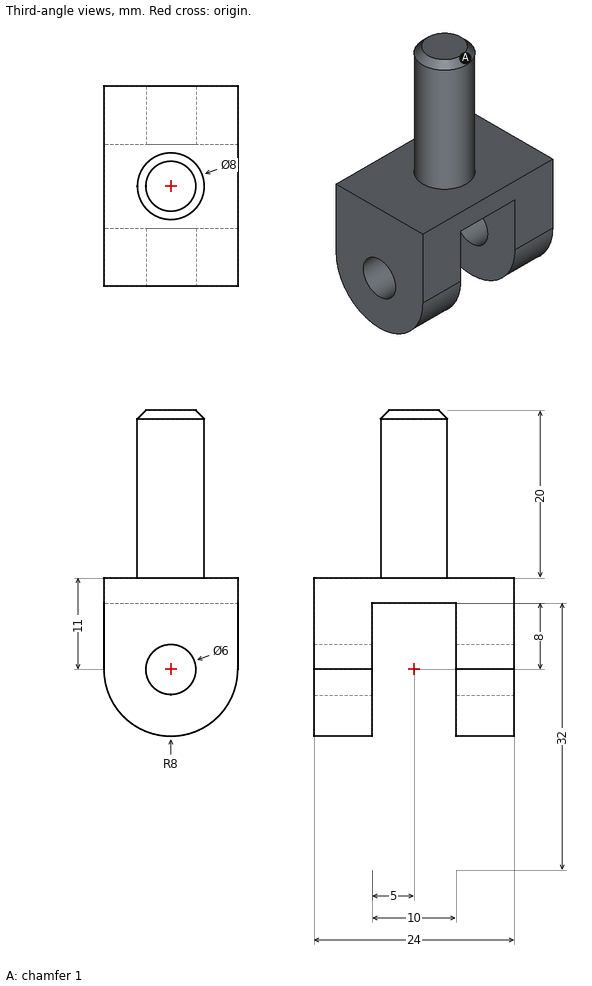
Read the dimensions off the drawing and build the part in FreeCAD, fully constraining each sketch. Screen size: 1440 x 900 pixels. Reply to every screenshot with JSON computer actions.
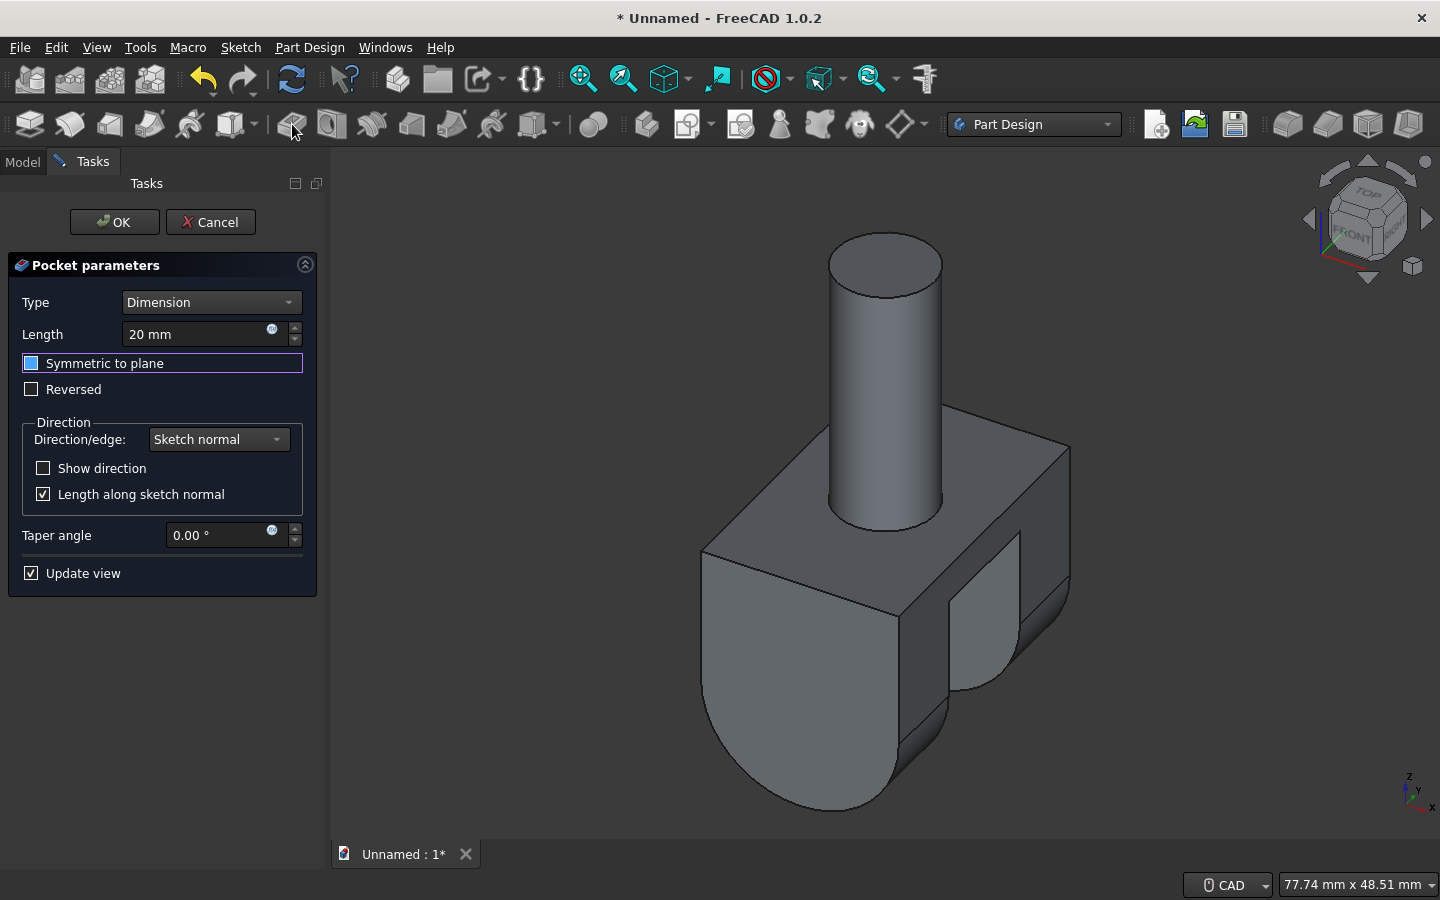
{"action": "left_click", "coordinate": [115, 222]}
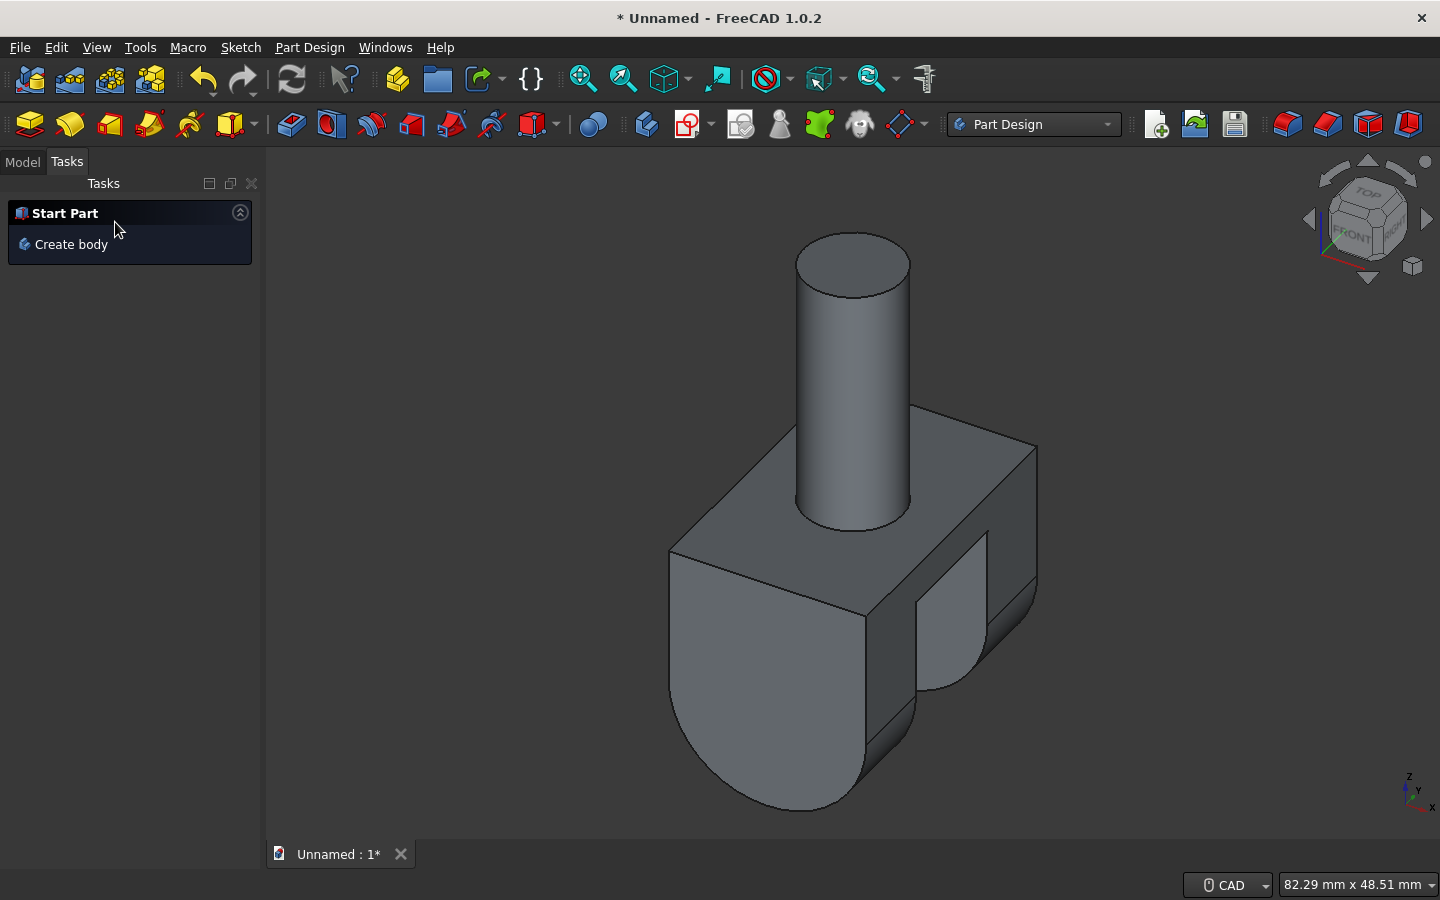
{"action": "left_click", "coordinate": [584, 80]}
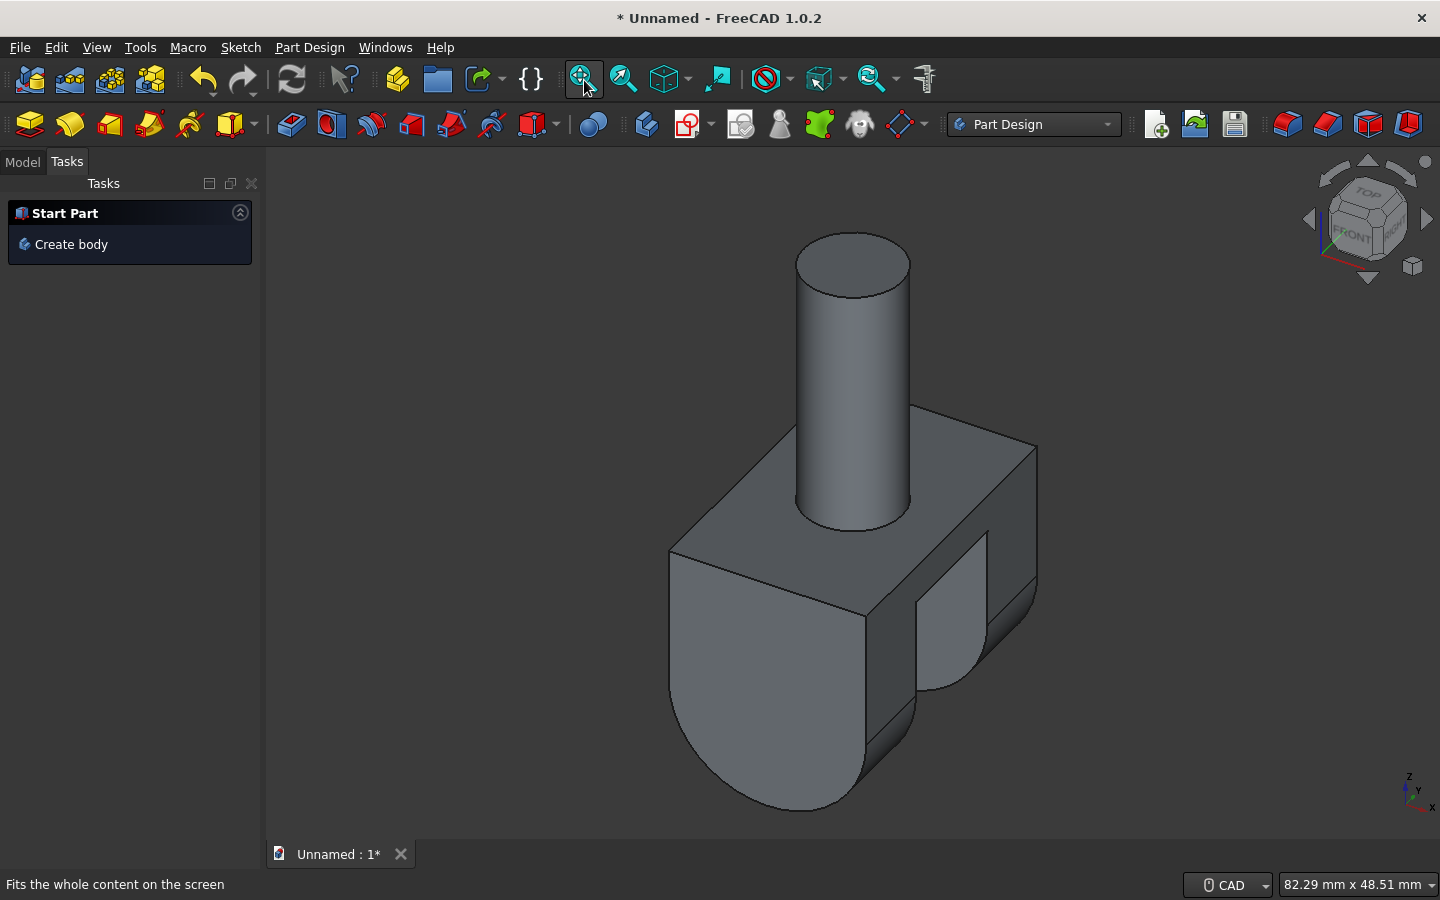
{"action": "left_click", "coordinate": [767, 694]}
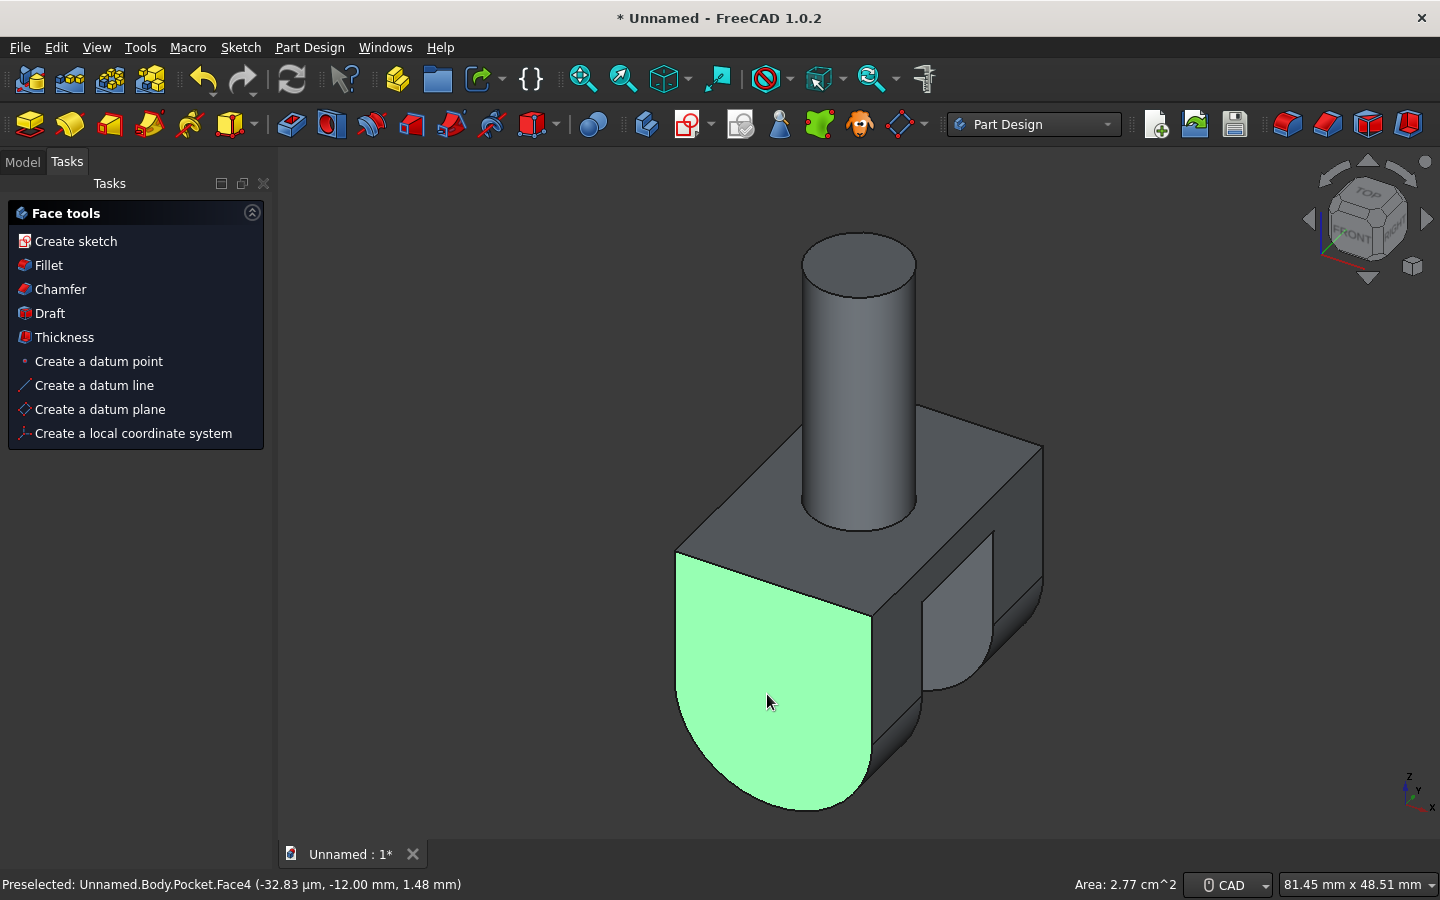
{"action": "left_click", "coordinate": [688, 124]}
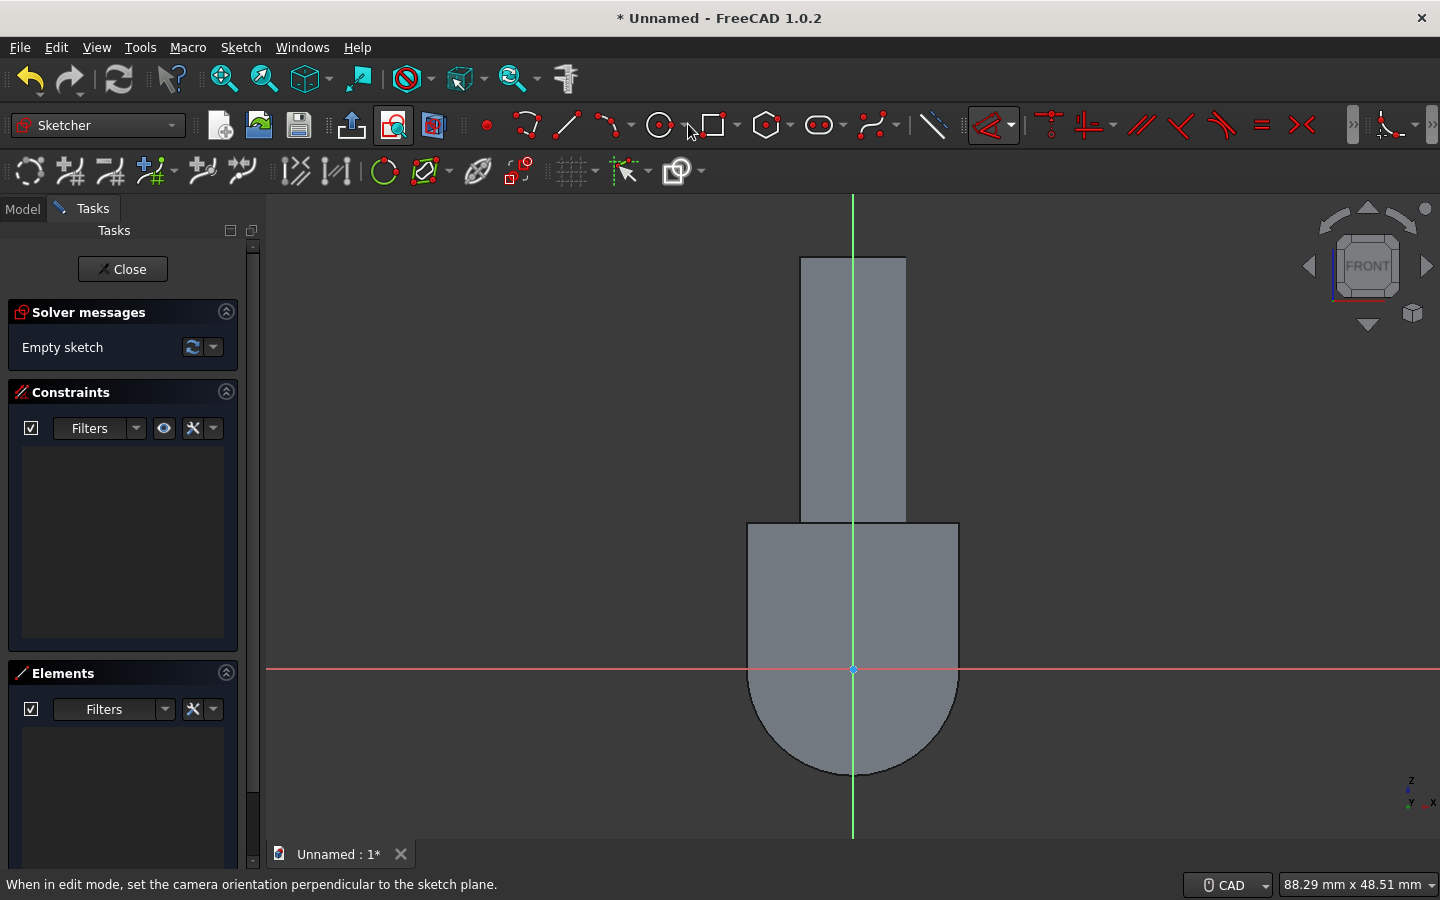
{"action": "scroll", "coordinate": [870, 708], "scroll_direction": "up", "scroll_amount": 8}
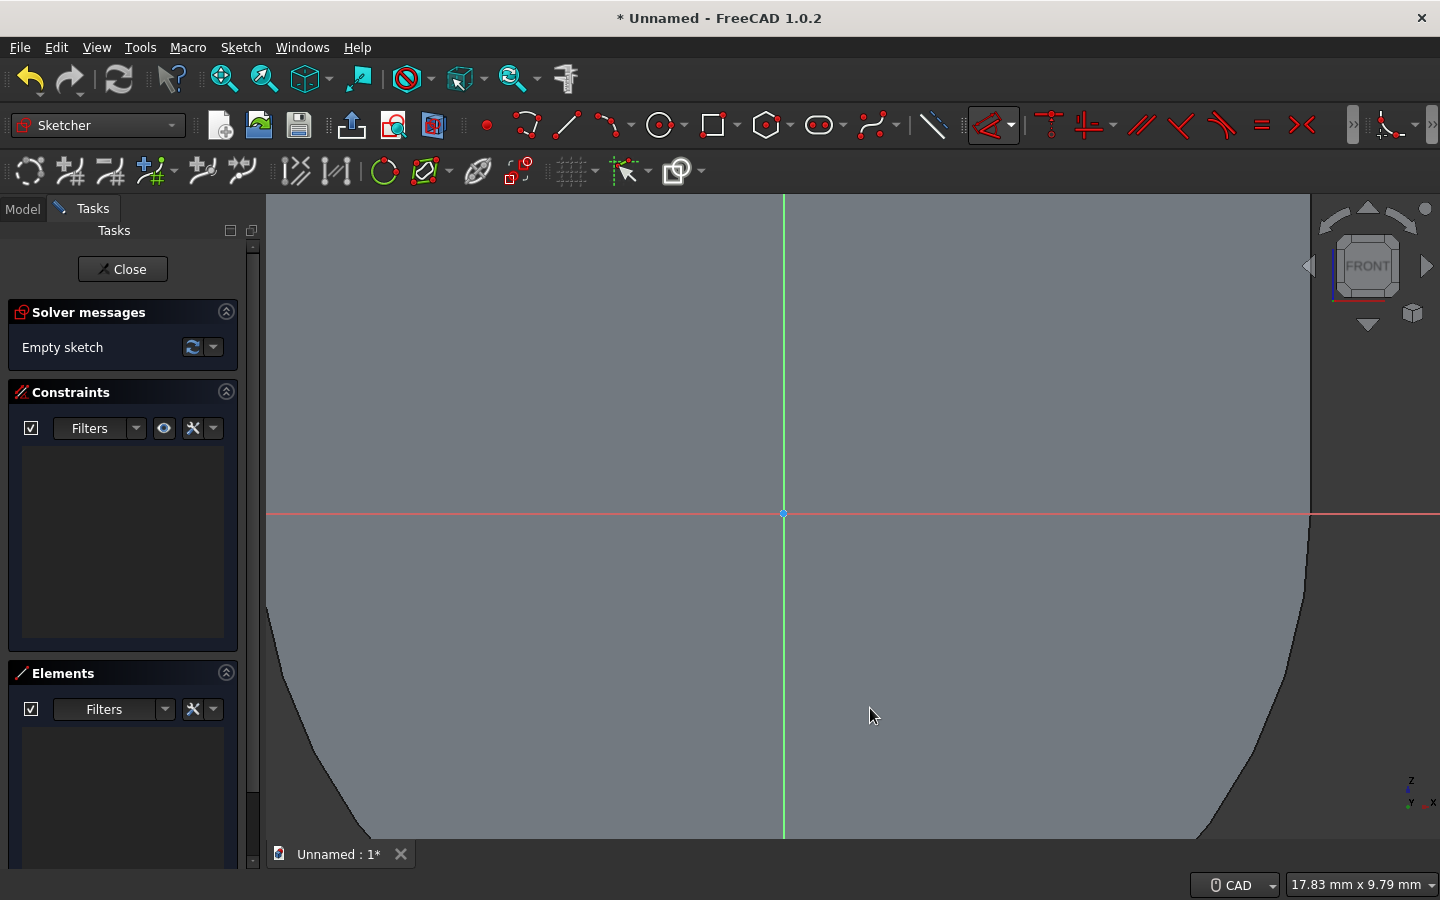
{"action": "left_click", "coordinate": [660, 126]}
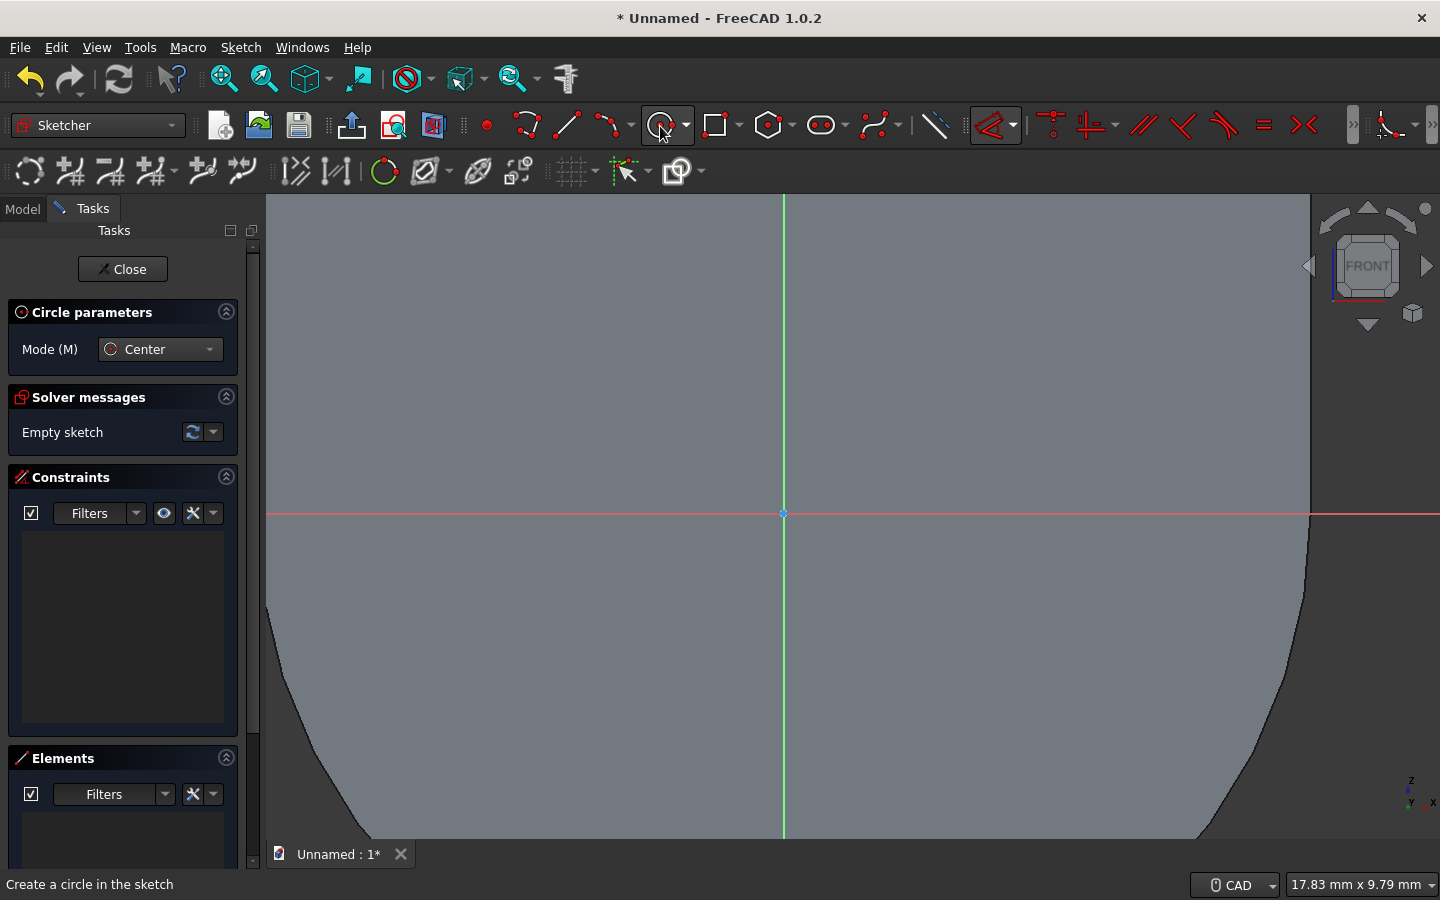
{"action": "left_click", "coordinate": [784, 514]}
{"action": "left_click", "coordinate": [923, 374]}
{"action": "key", "text": "Escape"}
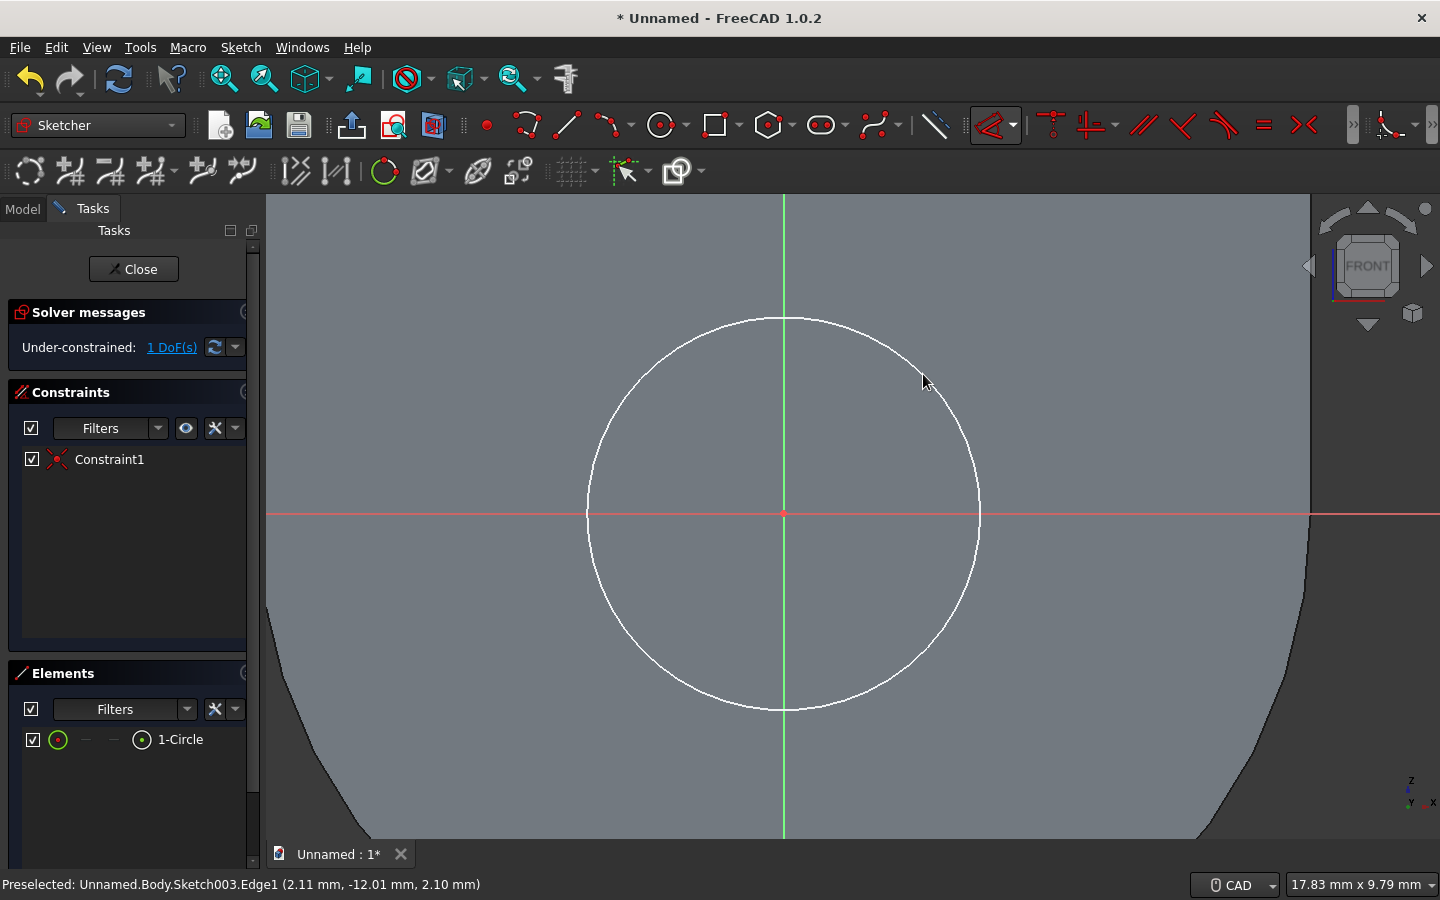
{"action": "left_click", "coordinate": [922, 374]}